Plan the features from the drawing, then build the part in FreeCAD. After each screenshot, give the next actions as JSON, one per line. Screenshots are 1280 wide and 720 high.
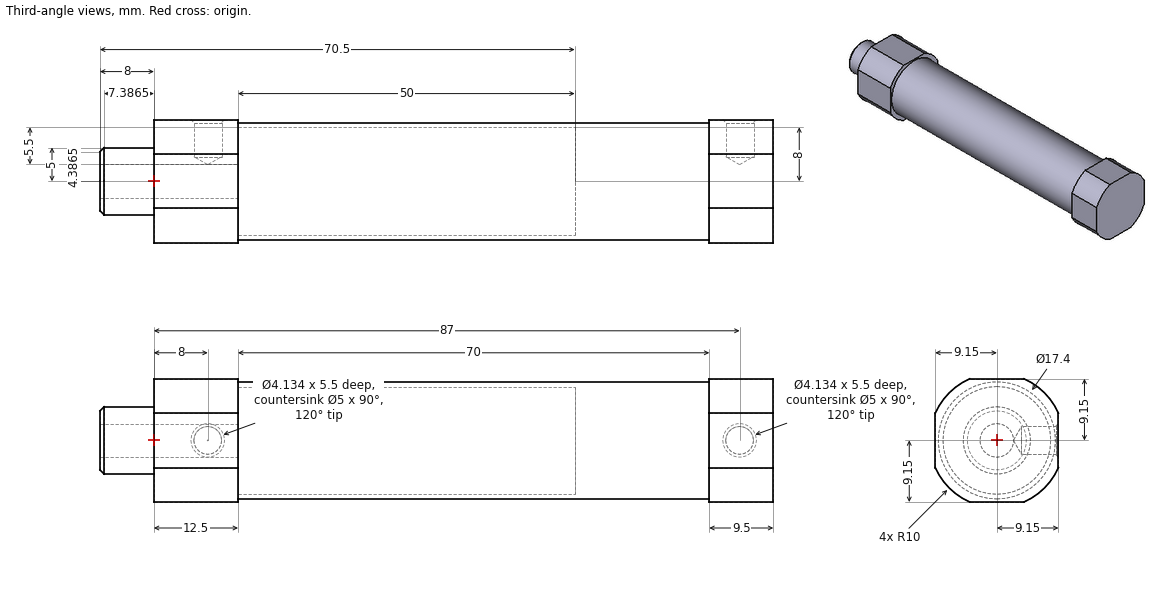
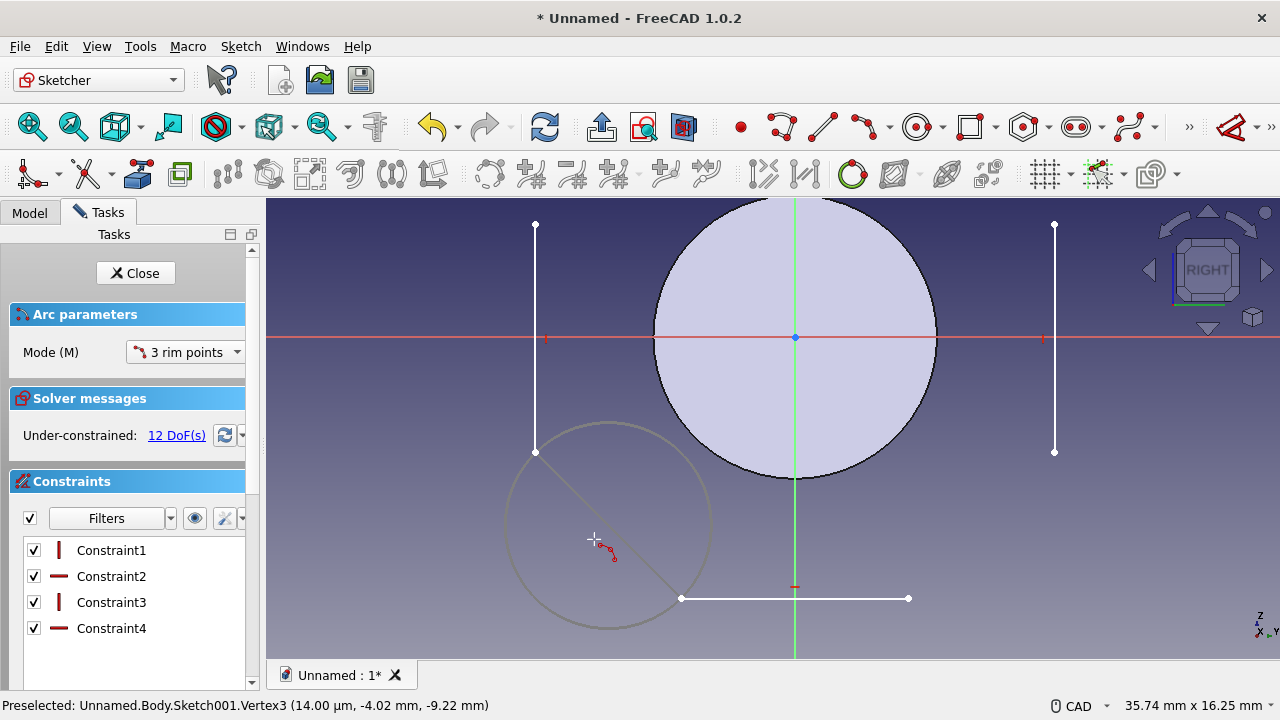
{"action": "left_click", "coordinate": [595, 538]}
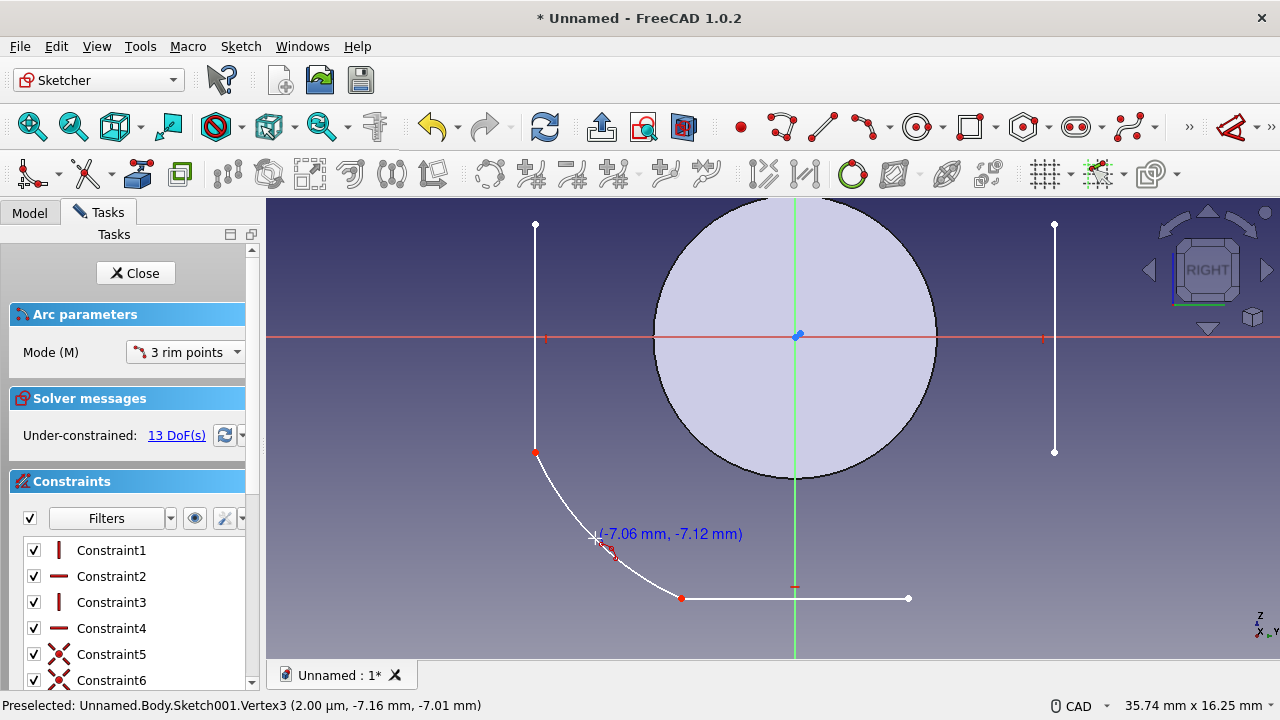
{"action": "left_click", "coordinate": [909, 599]}
{"action": "left_click", "coordinate": [1055, 453]}
{"action": "left_click", "coordinate": [996, 538]}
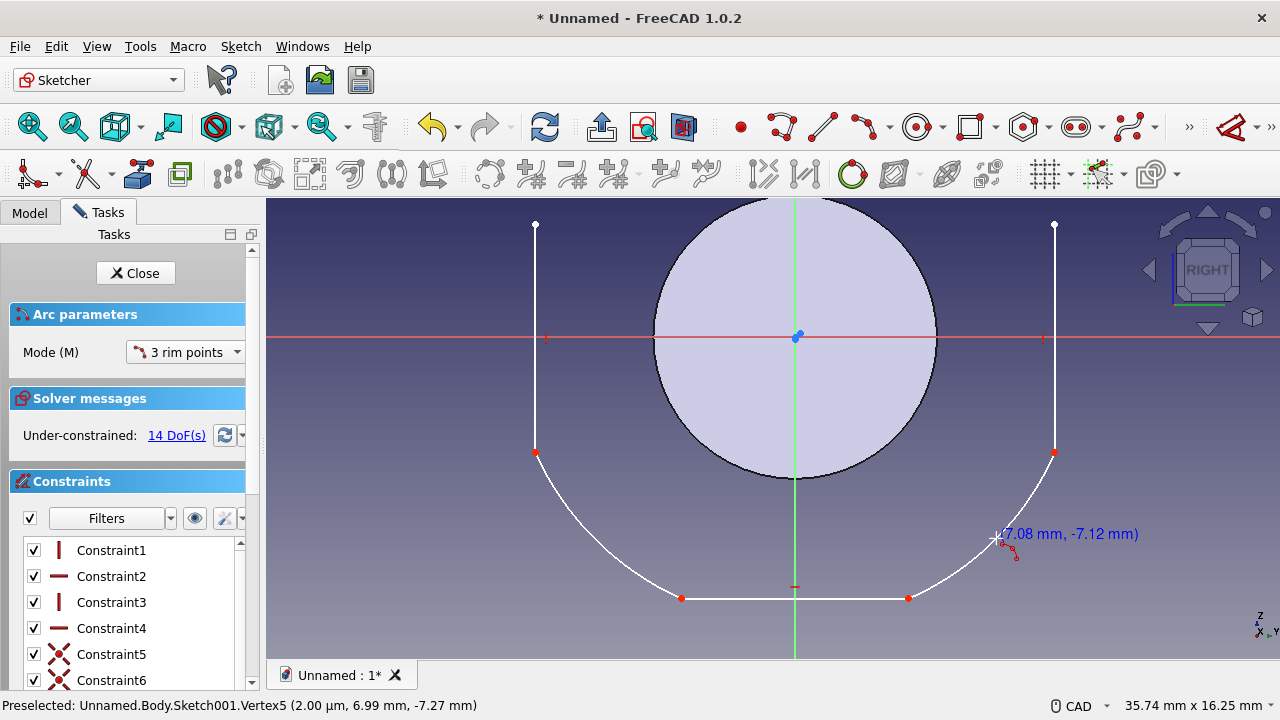
{"action": "scroll", "coordinate": [594, 540], "scroll_direction": "down", "scroll_amount": 3}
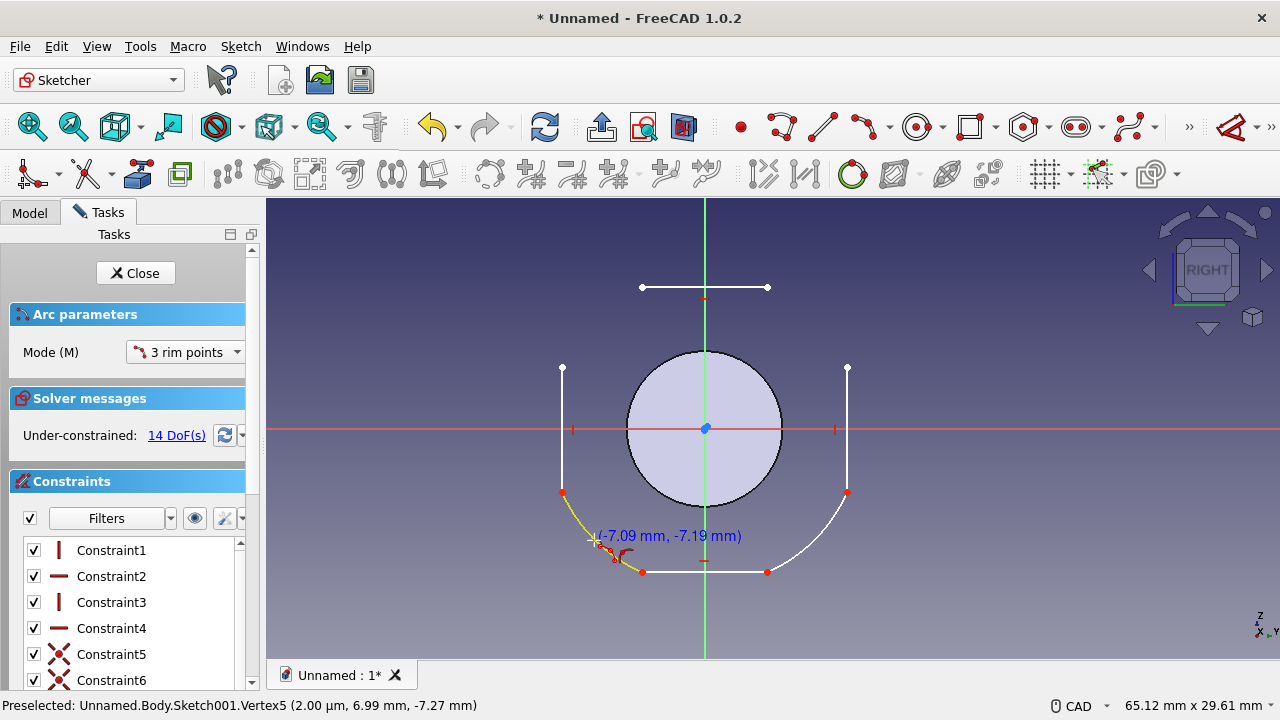
{"action": "left_click", "coordinate": [847, 367]}
{"action": "left_click", "coordinate": [767, 287]}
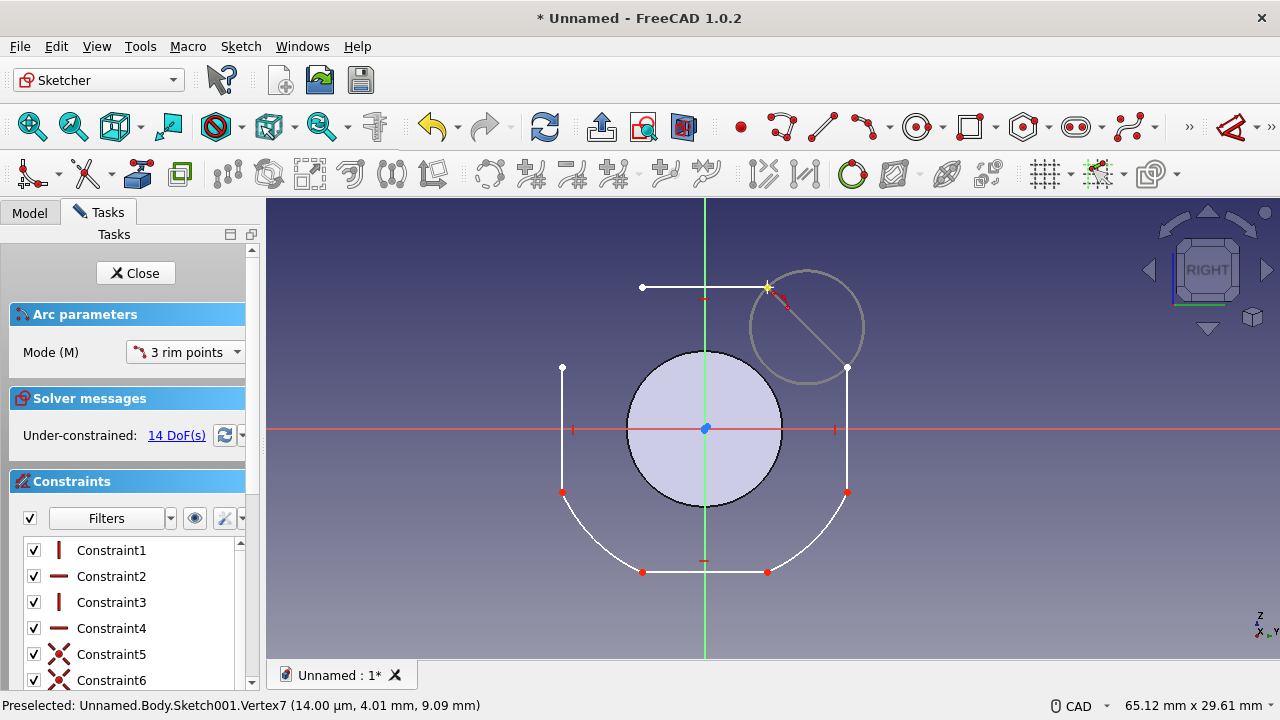
{"action": "scroll", "coordinate": [815, 319], "scroll_direction": "up", "scroll_amount": 3}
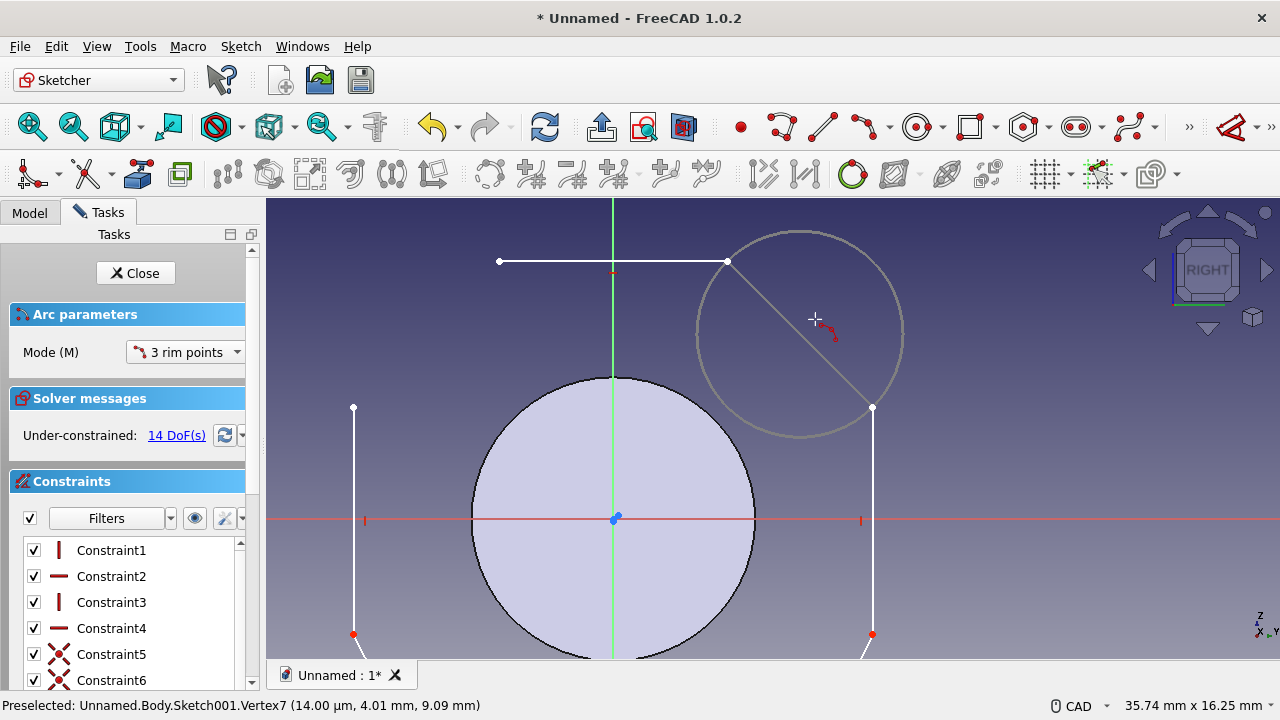
{"action": "left_click", "coordinate": [814, 319]}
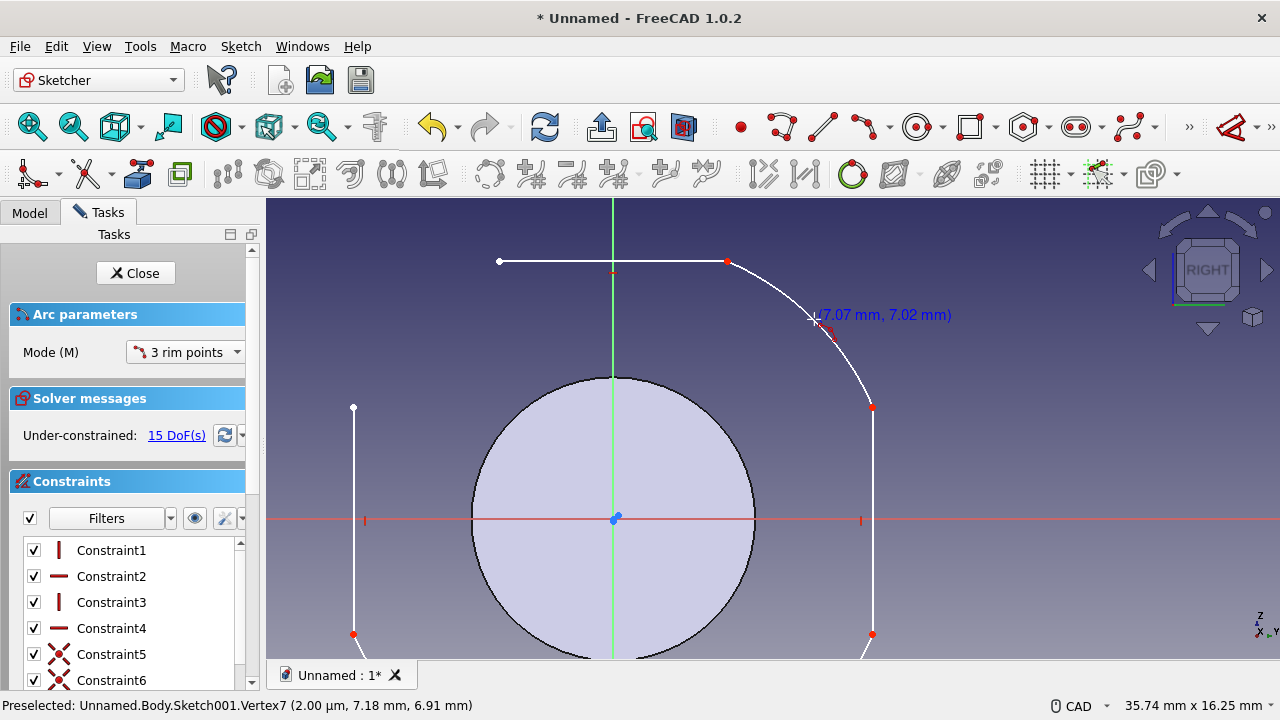
{"action": "left_click", "coordinate": [499, 261]}
{"action": "left_click", "coordinate": [354, 407]}
{"action": "left_click", "coordinate": [413, 319]}
{"action": "key", "text": "Escape"}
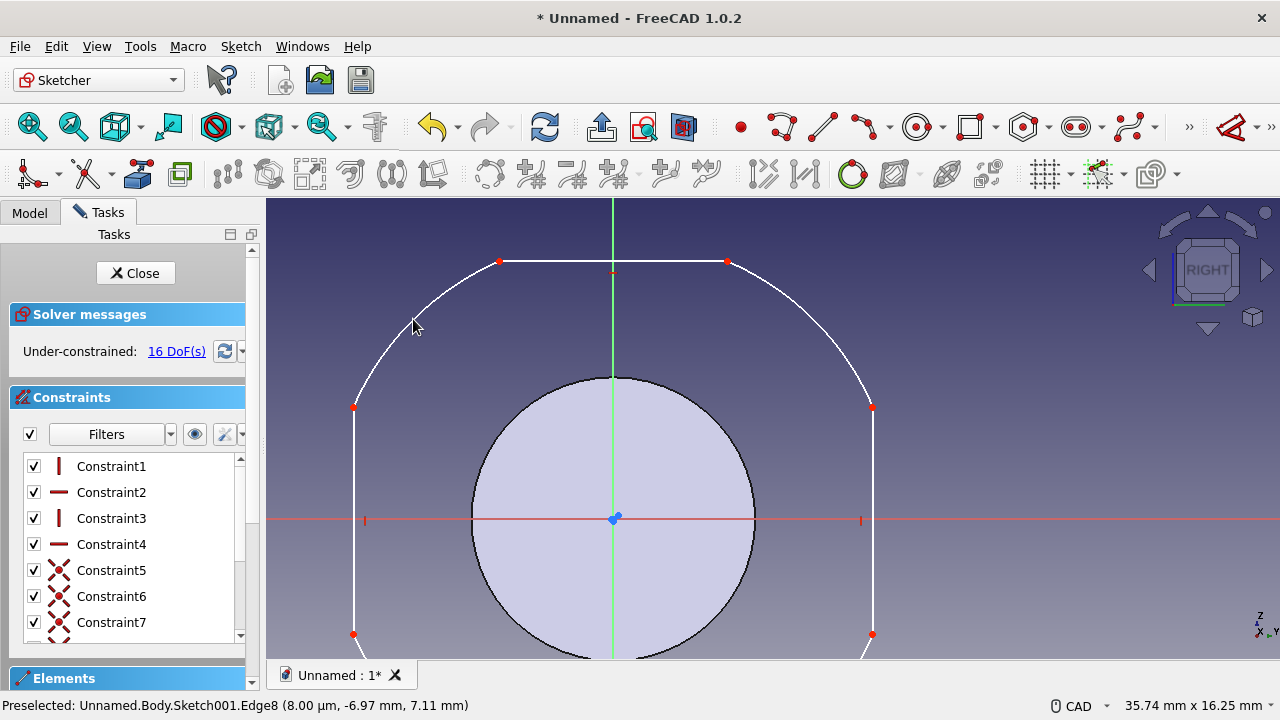
{"action": "scroll", "coordinate": [815, 318], "scroll_direction": "down", "scroll_amount": 3}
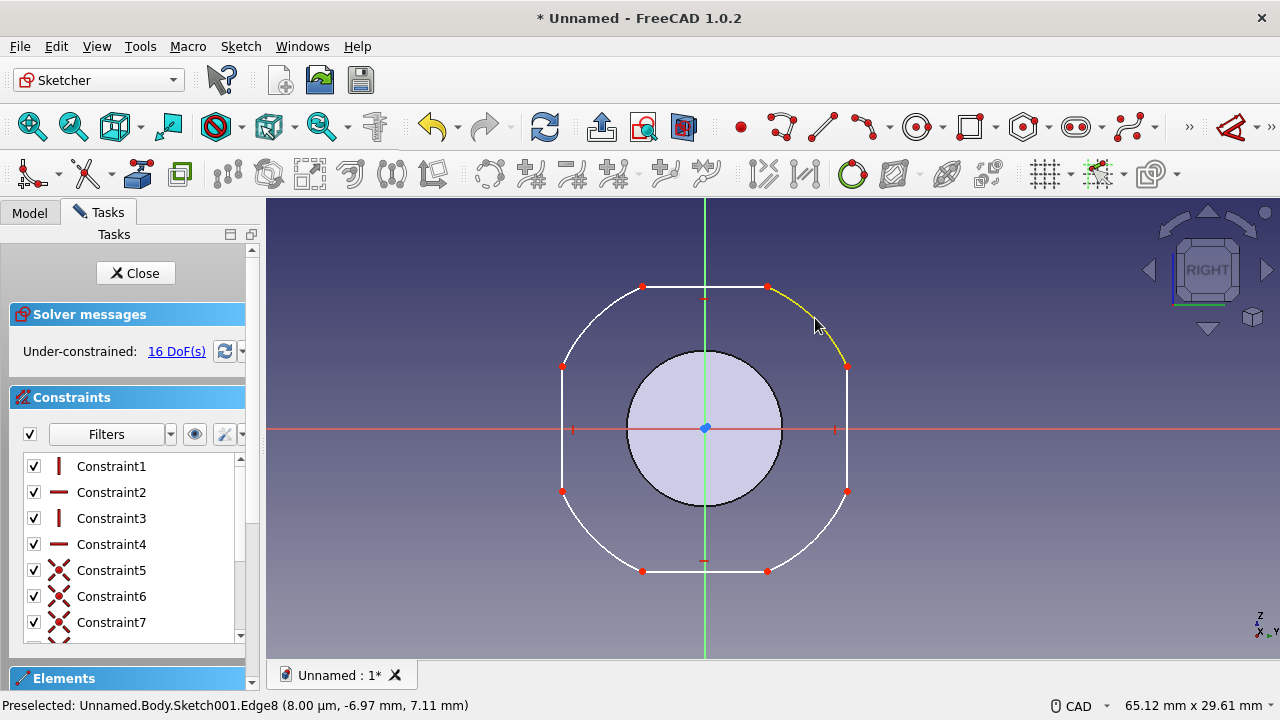
{"action": "left_click", "coordinate": [580, 522]}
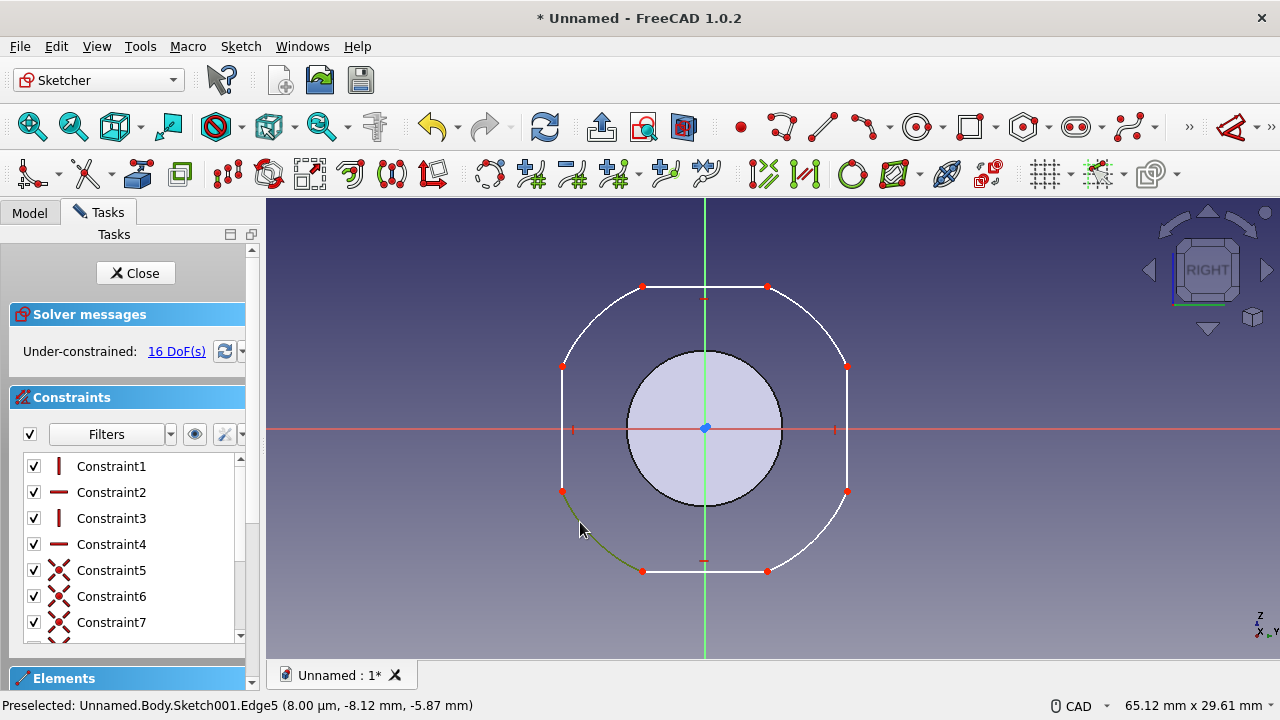
{"action": "left_click", "coordinate": [797, 555]}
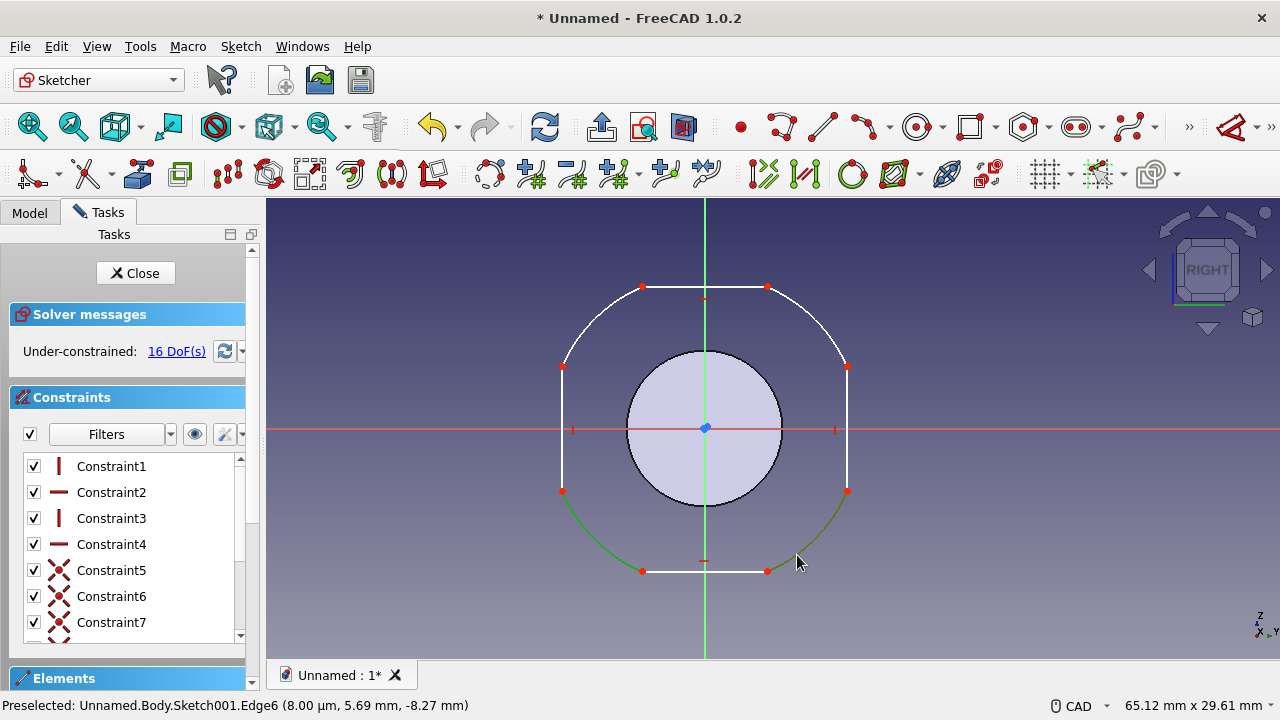
{"action": "key", "text": "c"}